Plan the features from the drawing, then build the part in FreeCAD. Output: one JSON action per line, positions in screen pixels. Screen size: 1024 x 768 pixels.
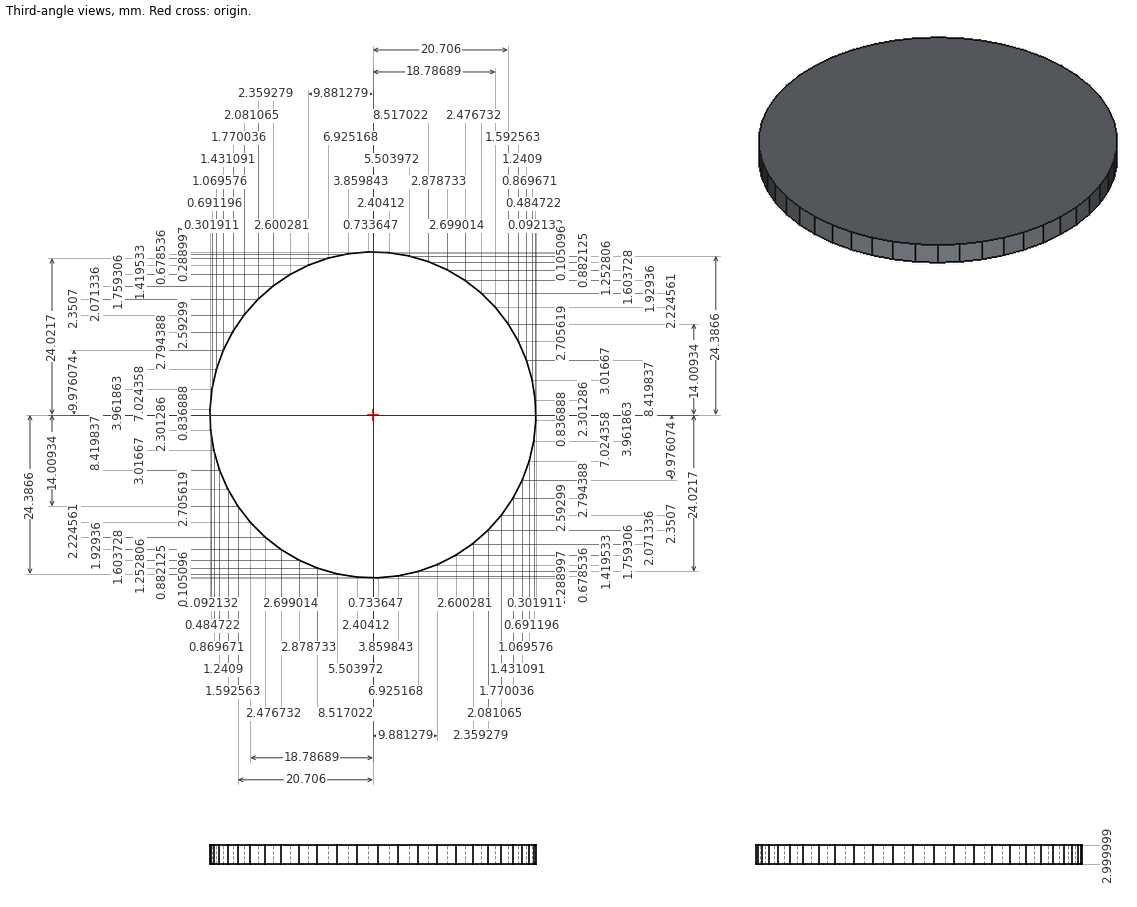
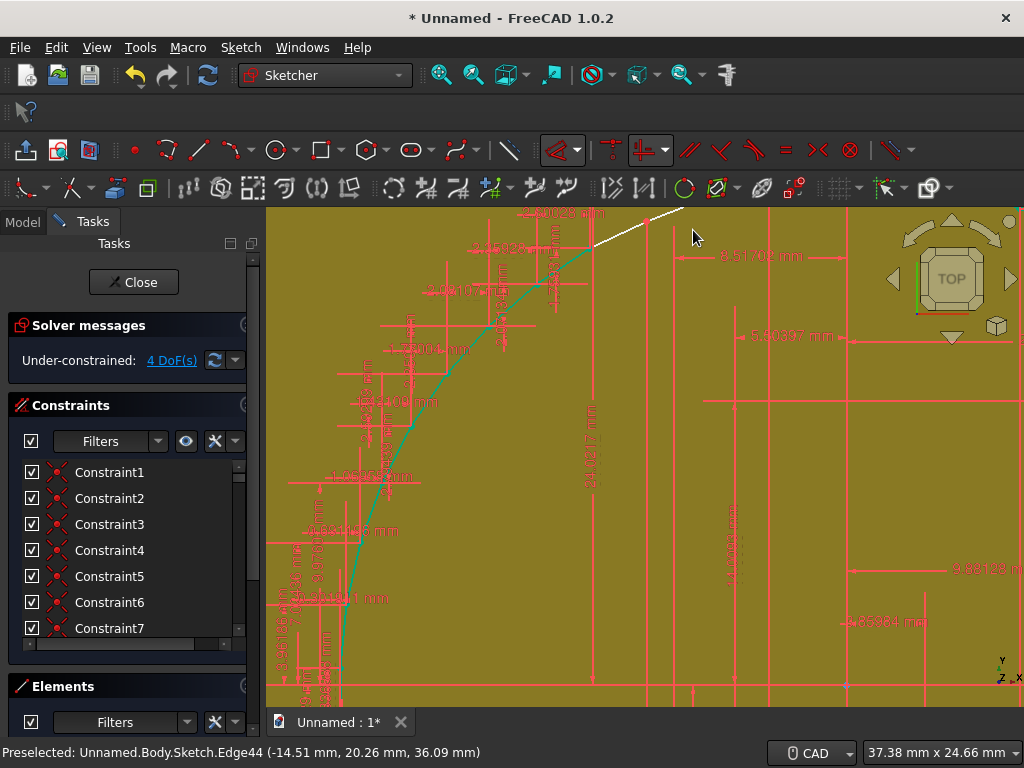
{"action": "scroll", "coordinate": [607, 240], "scroll_direction": "up", "scroll_amount": 2}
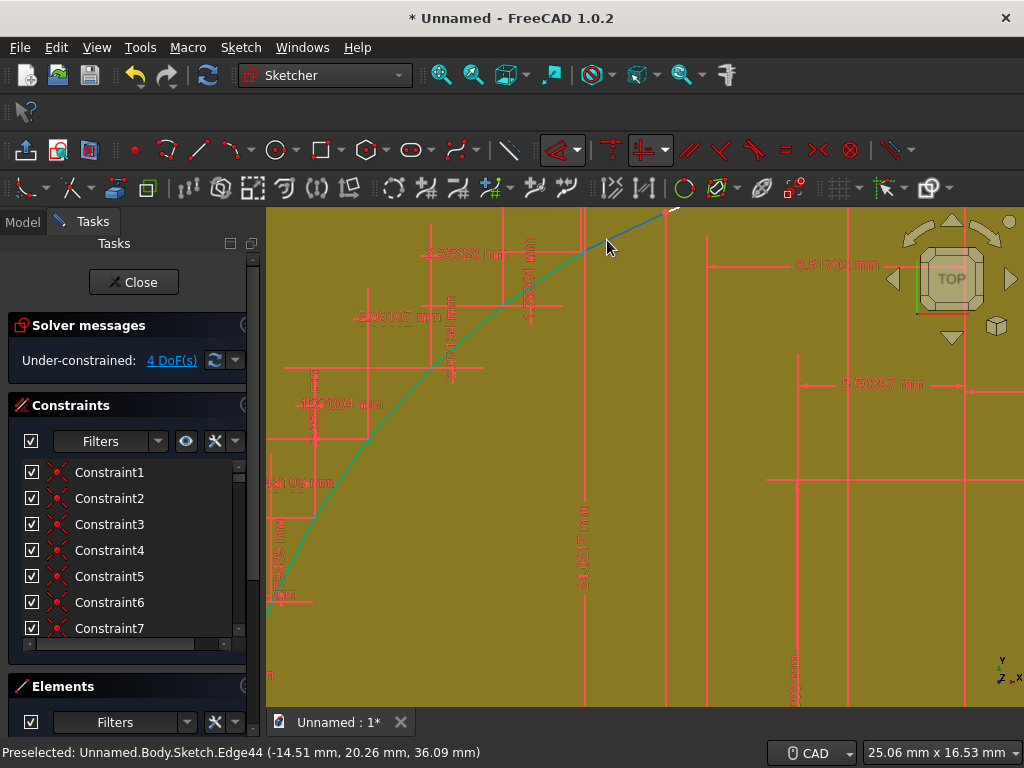
{"action": "left_click", "coordinate": [607, 241]}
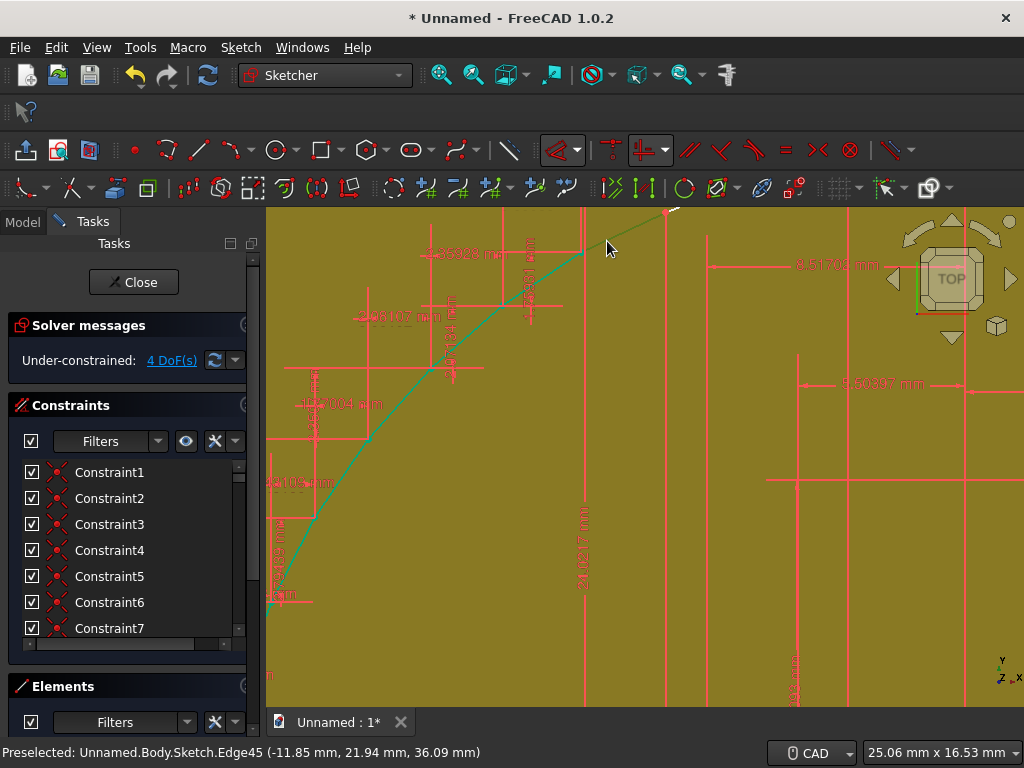
{"action": "left_click", "coordinate": [580, 150]}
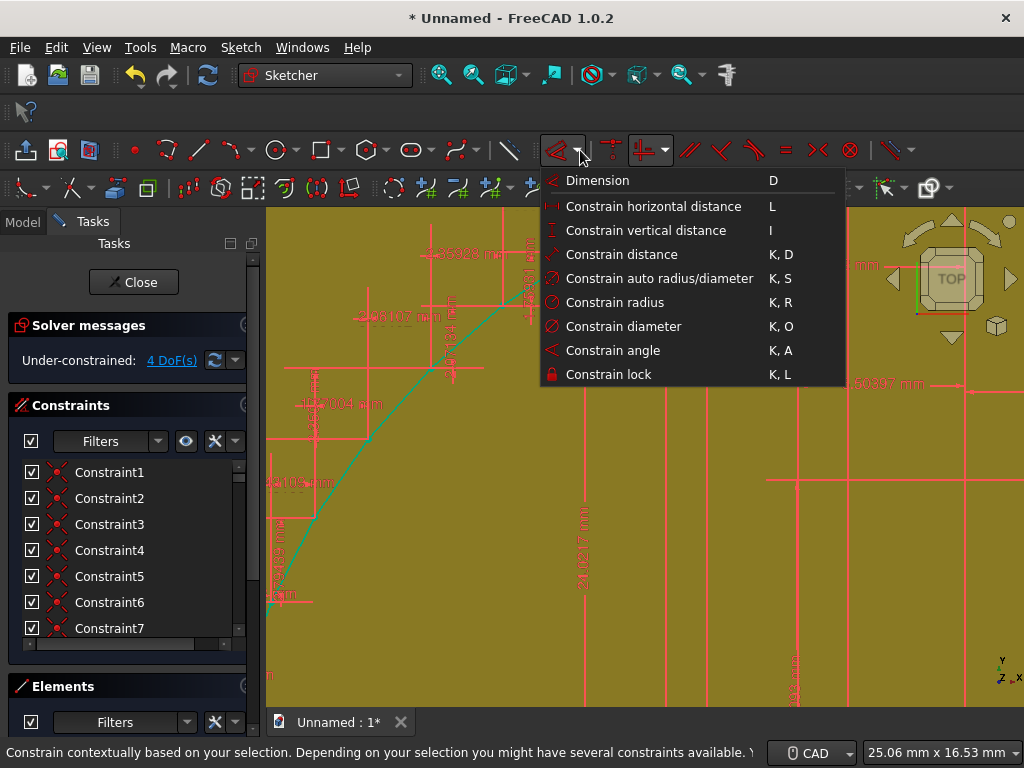
{"action": "left_click", "coordinate": [693, 230]}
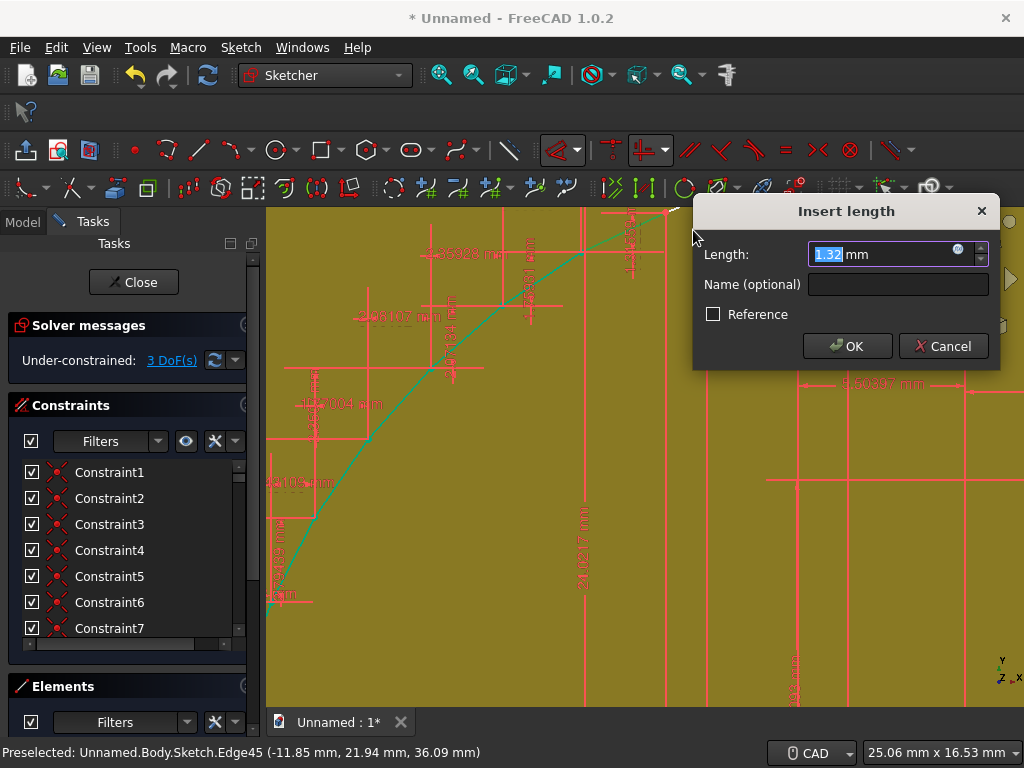
{"action": "type", "text": "1.419533"}
{"action": "key", "text": "Return"}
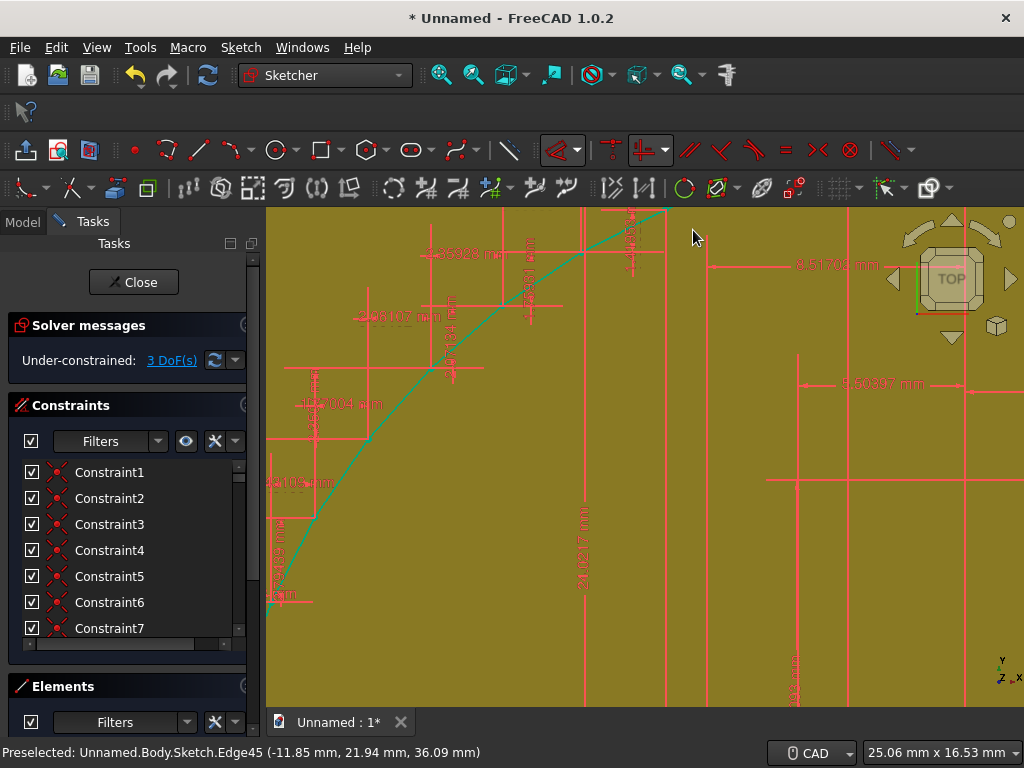
{"action": "scroll", "coordinate": [478, 344], "scroll_direction": "down", "scroll_amount": 8}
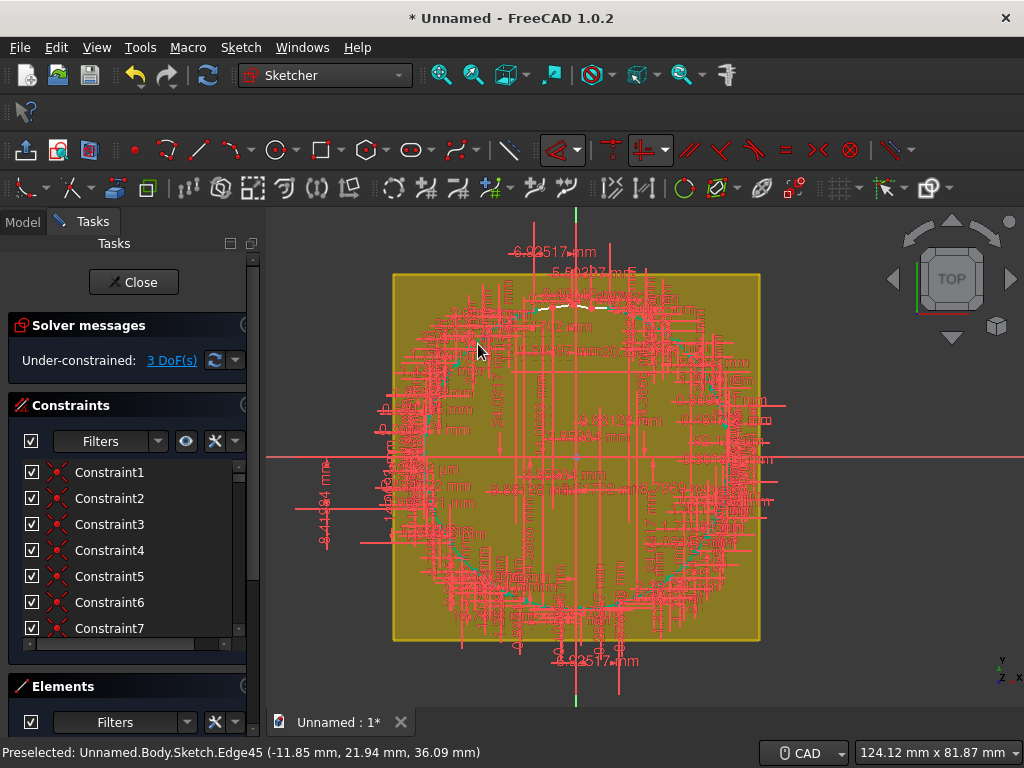
{"action": "scroll", "coordinate": [540, 310], "scroll_direction": "up", "scroll_amount": 12}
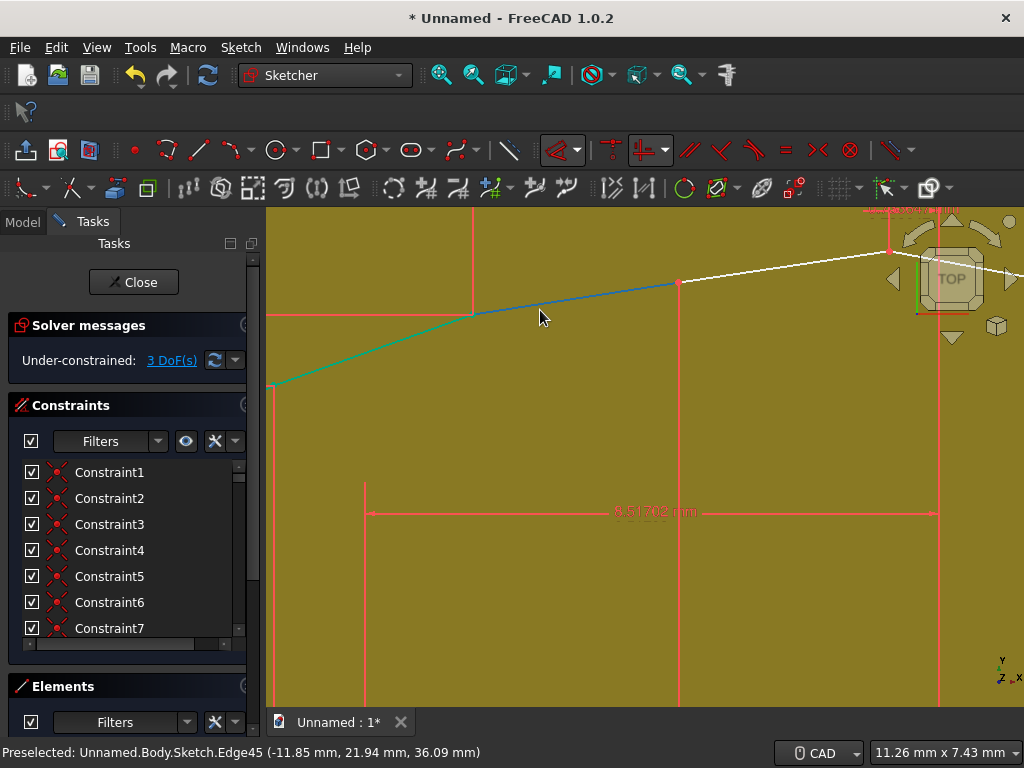
{"action": "left_click", "coordinate": [534, 305]}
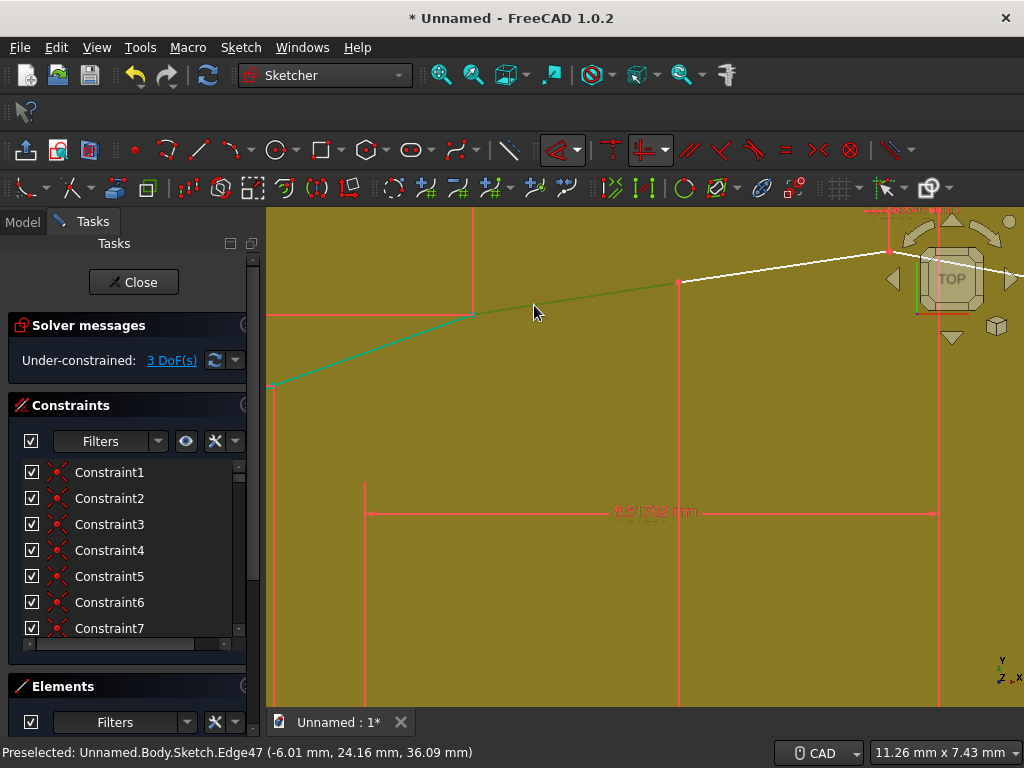
{"action": "left_click", "coordinate": [580, 150]}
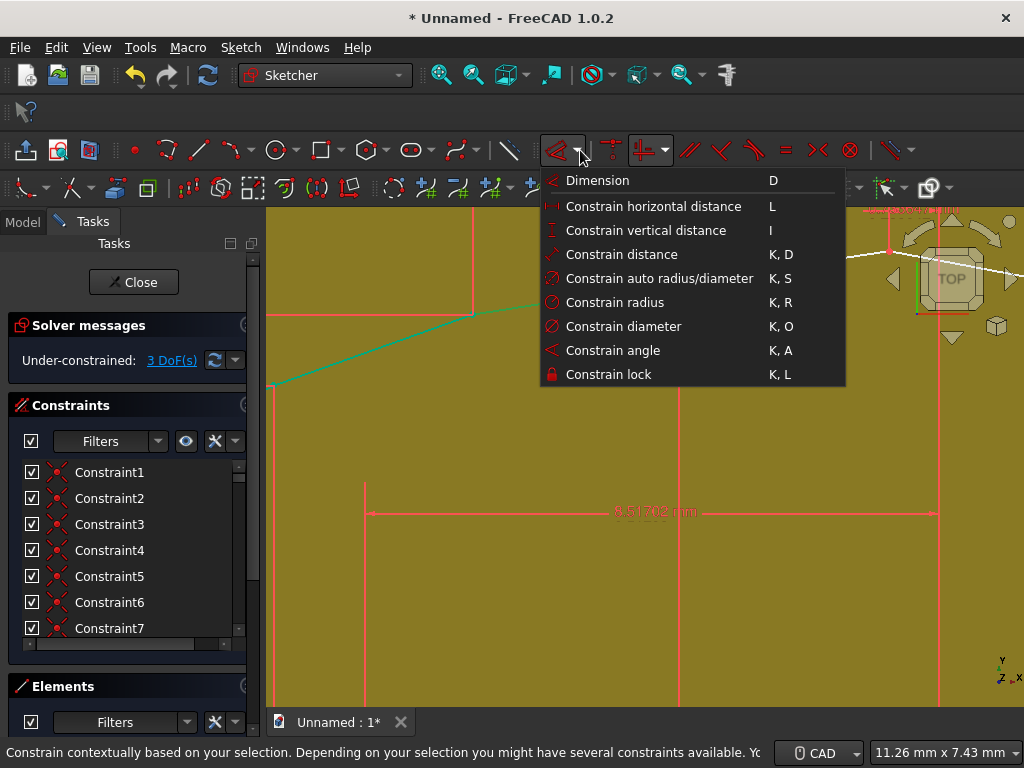
{"action": "left_click", "coordinate": [693, 230]}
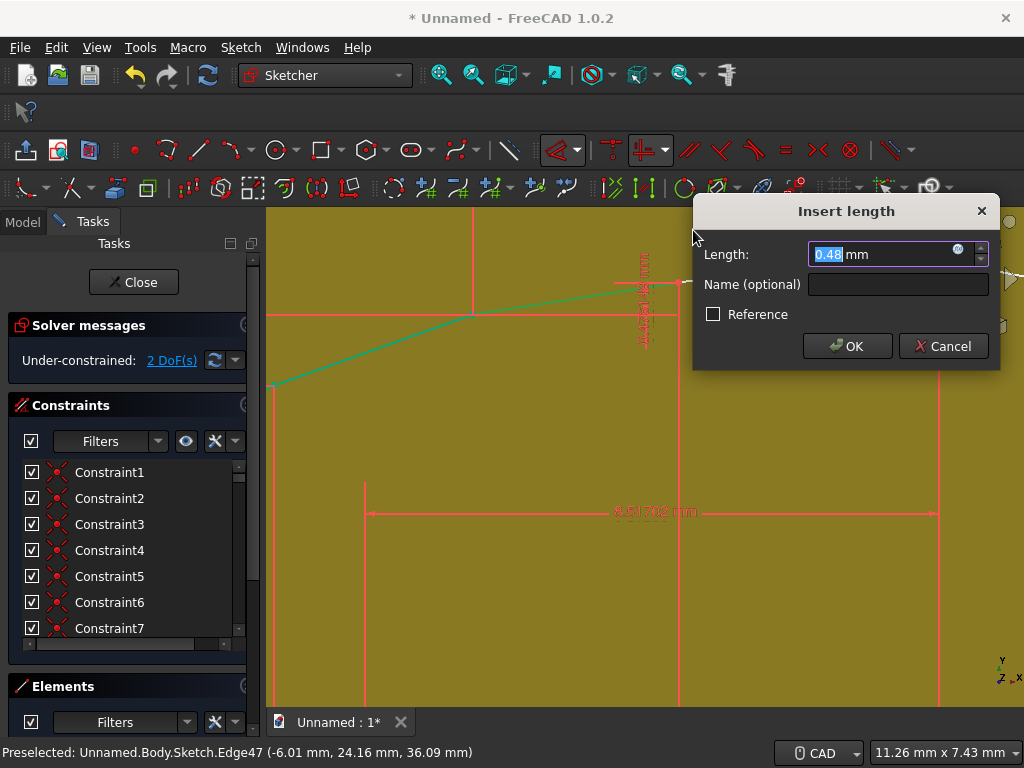
{"action": "type", "text": "0.678536"}
{"action": "key", "text": "Return"}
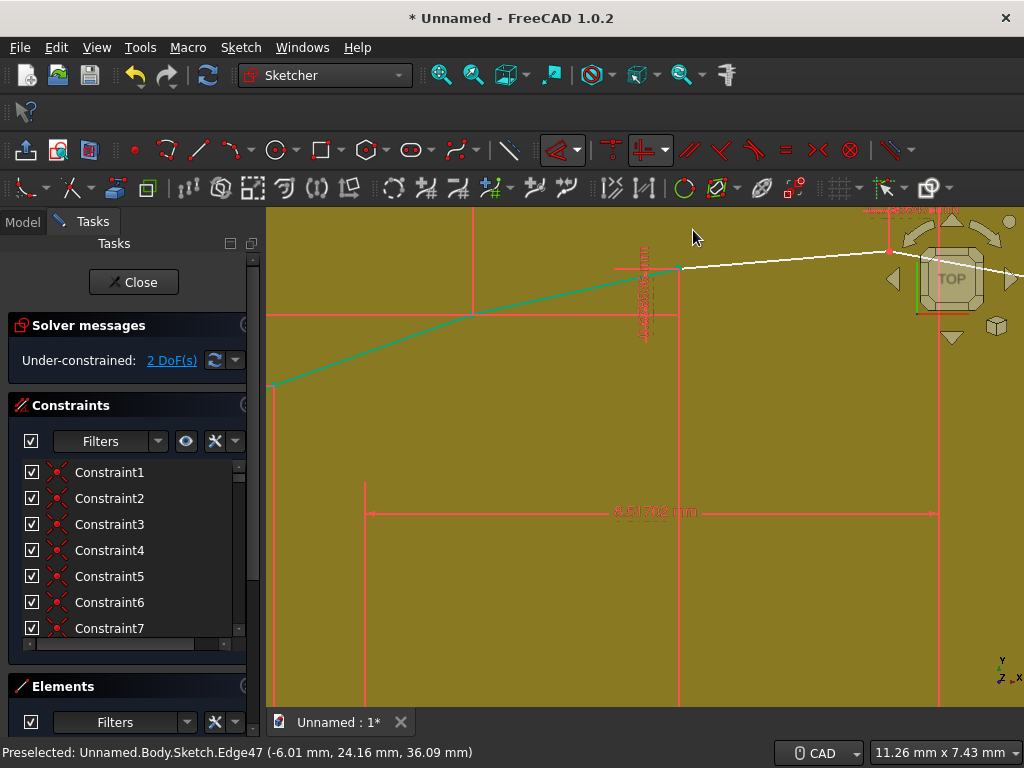
{"action": "scroll", "coordinate": [742, 264], "scroll_direction": "up", "scroll_amount": 4}